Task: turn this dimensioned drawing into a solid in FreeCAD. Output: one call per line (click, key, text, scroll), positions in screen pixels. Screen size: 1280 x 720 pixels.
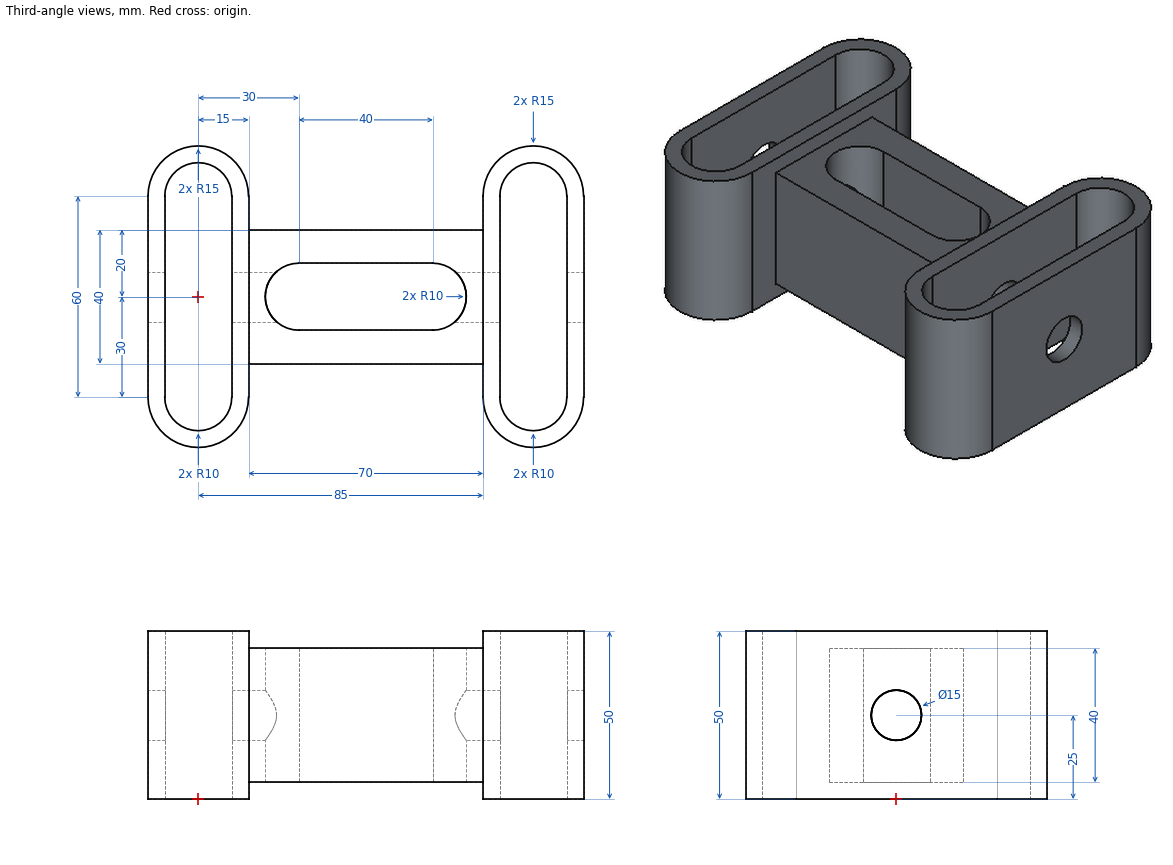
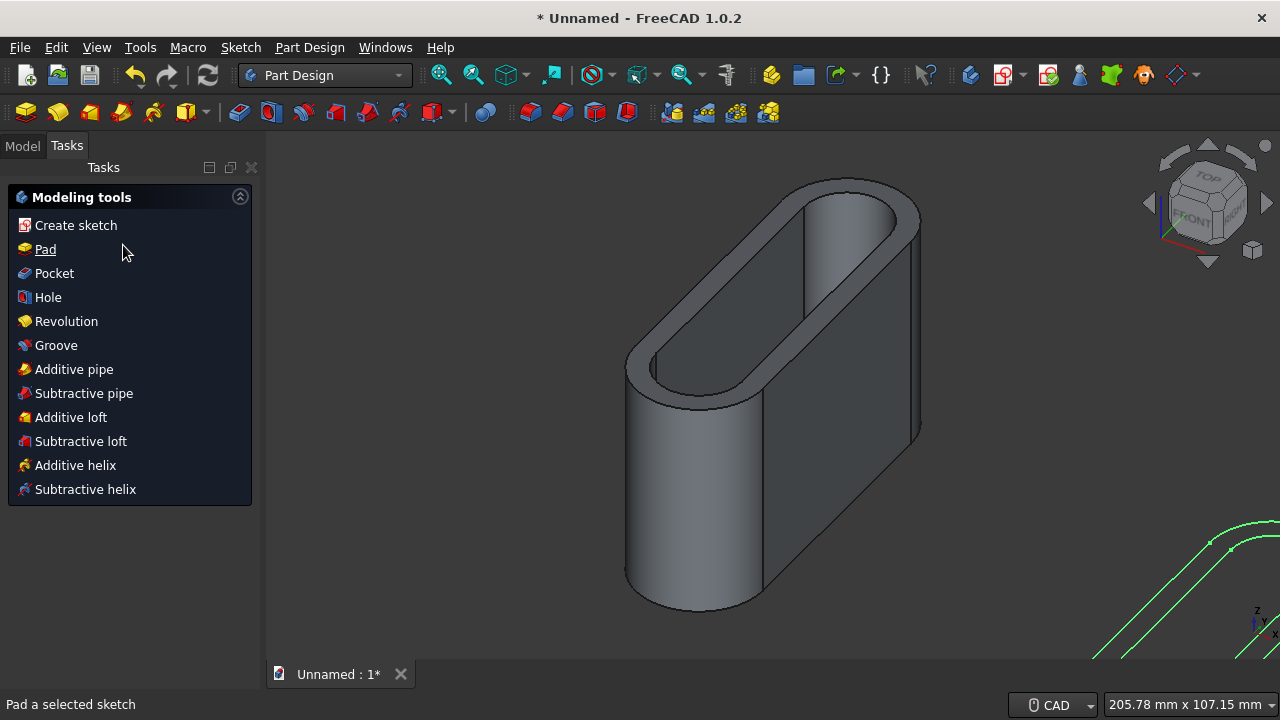
click(26, 112)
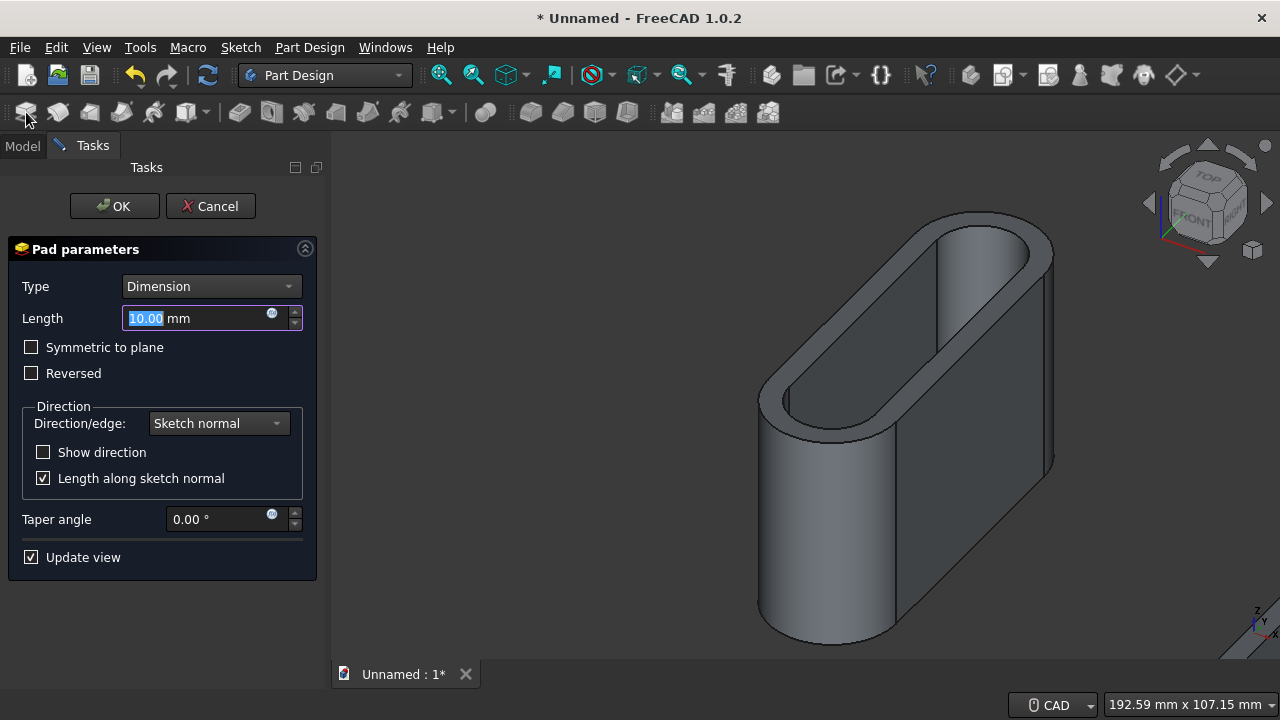
text(50)
key(Tab)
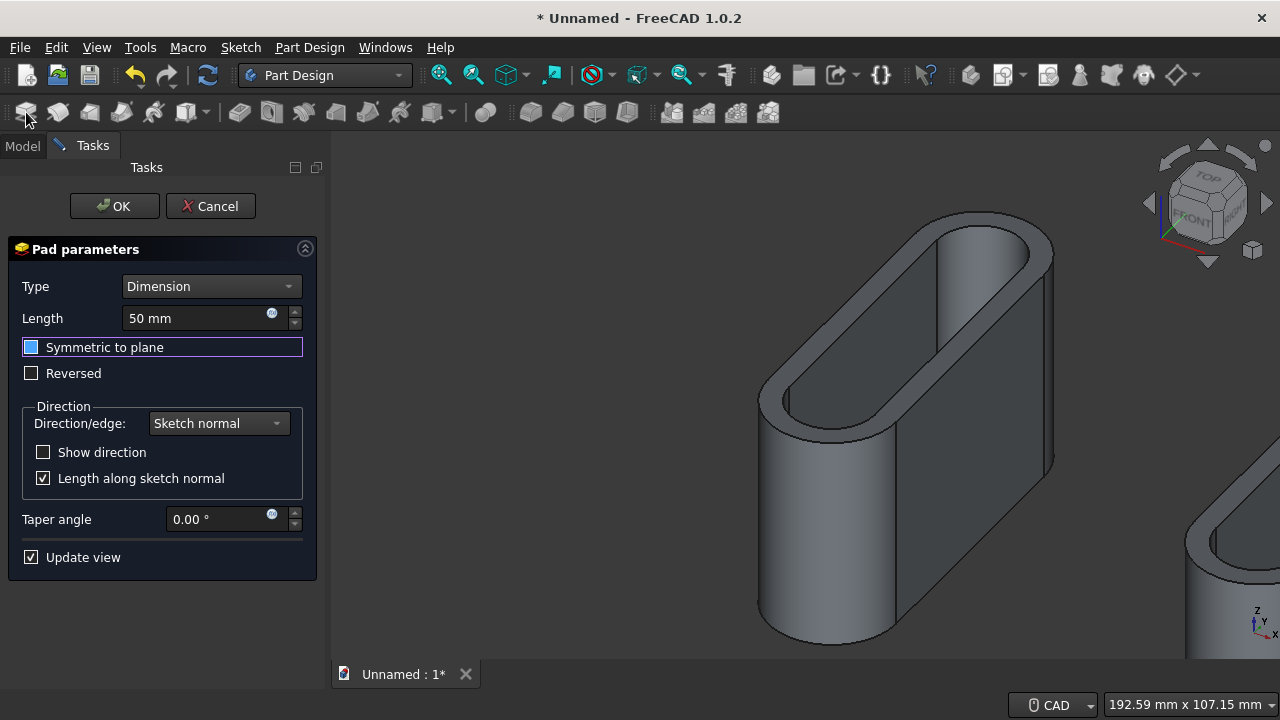
click(115, 206)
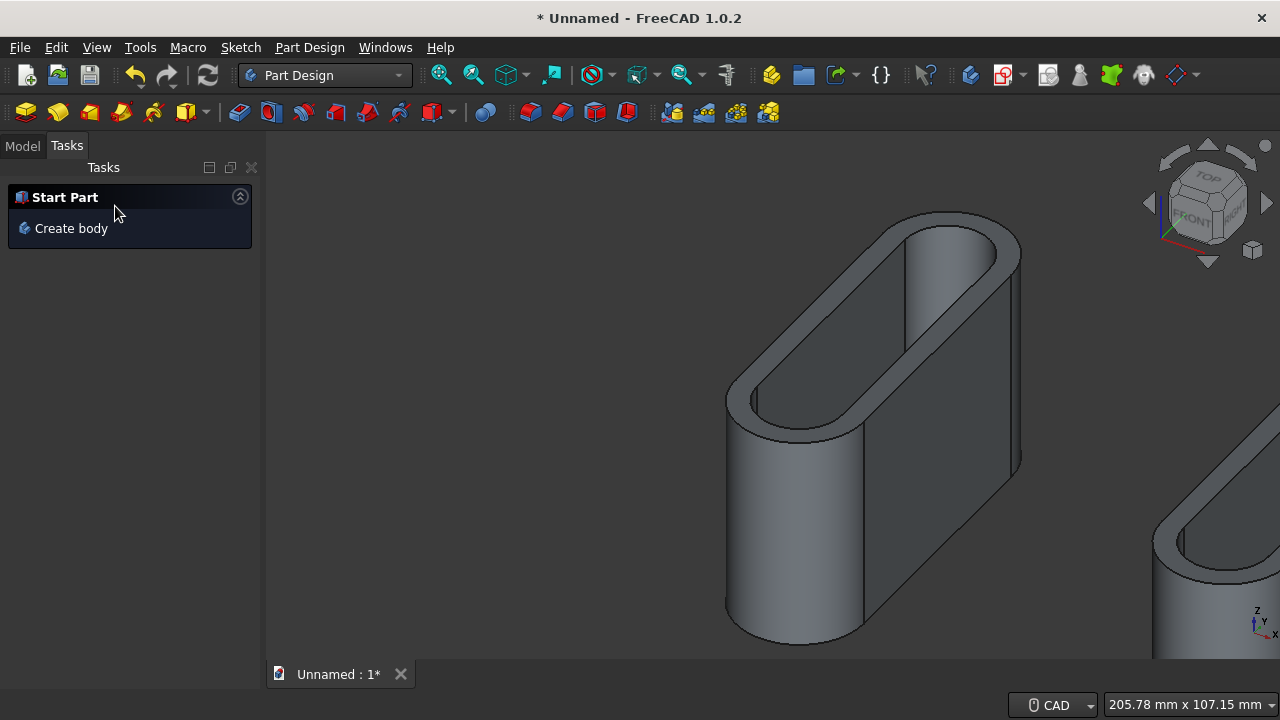
click(442, 76)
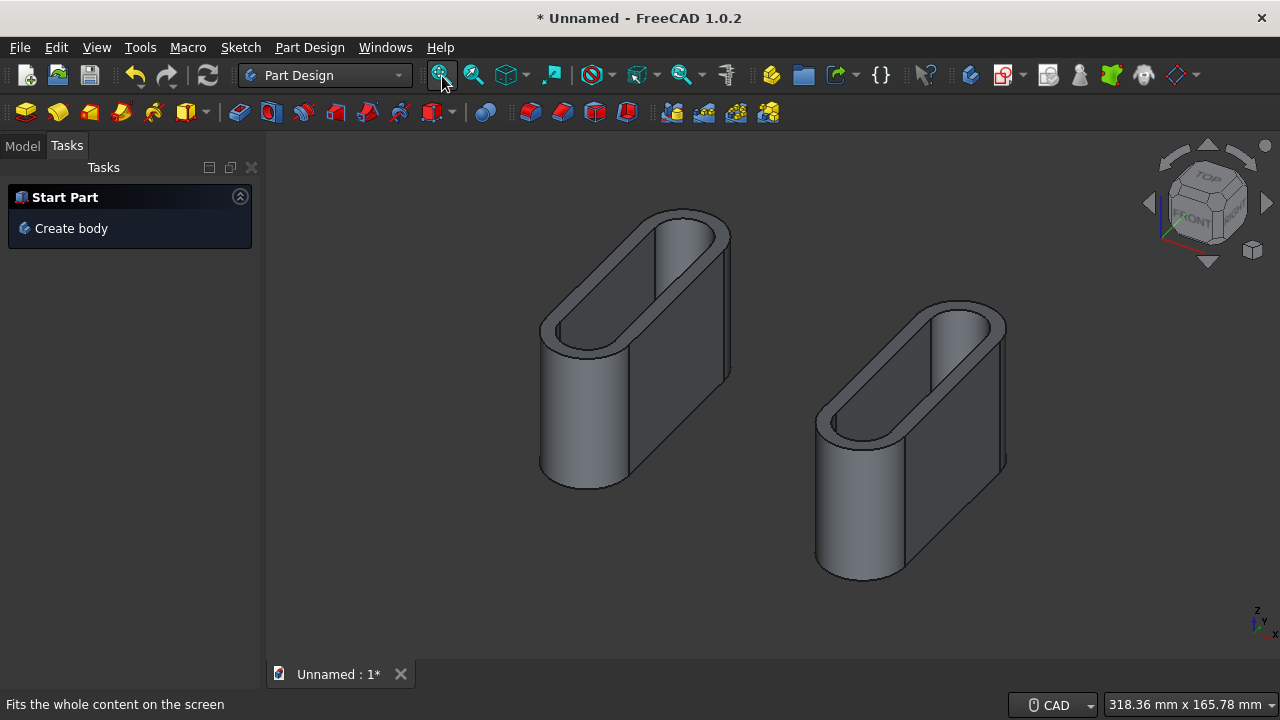
click(23, 145)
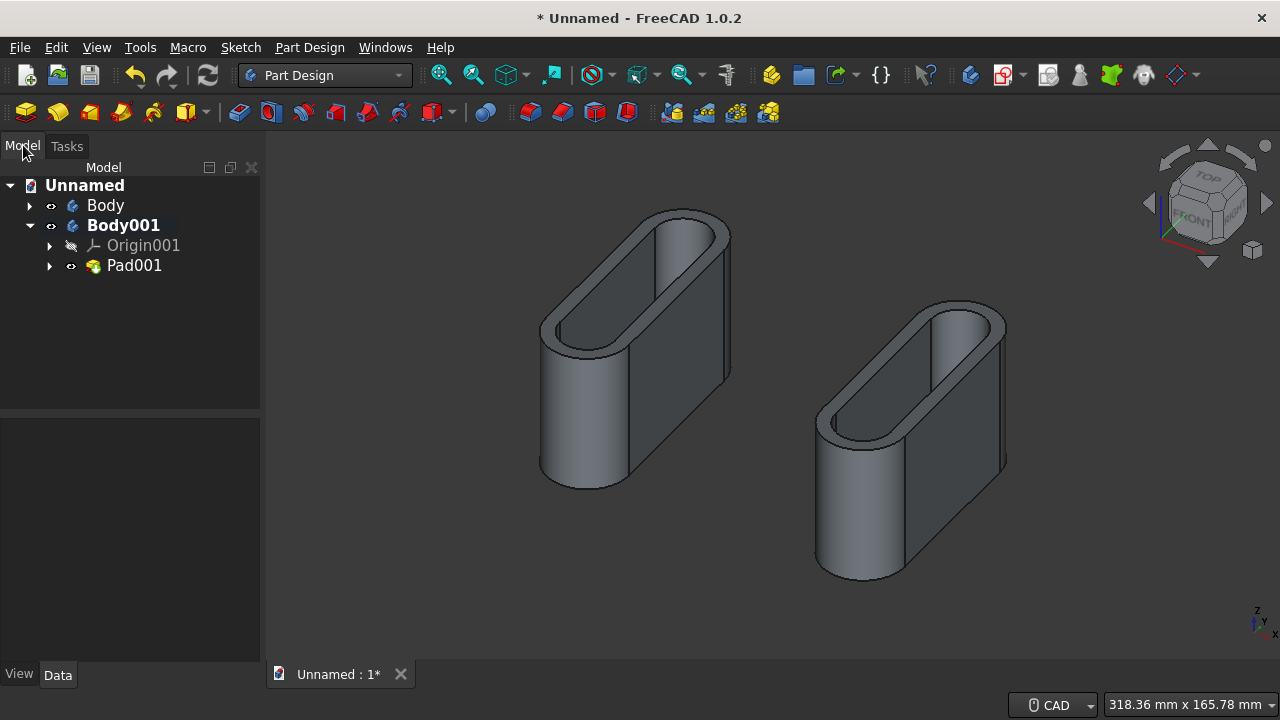
double_click(96, 206)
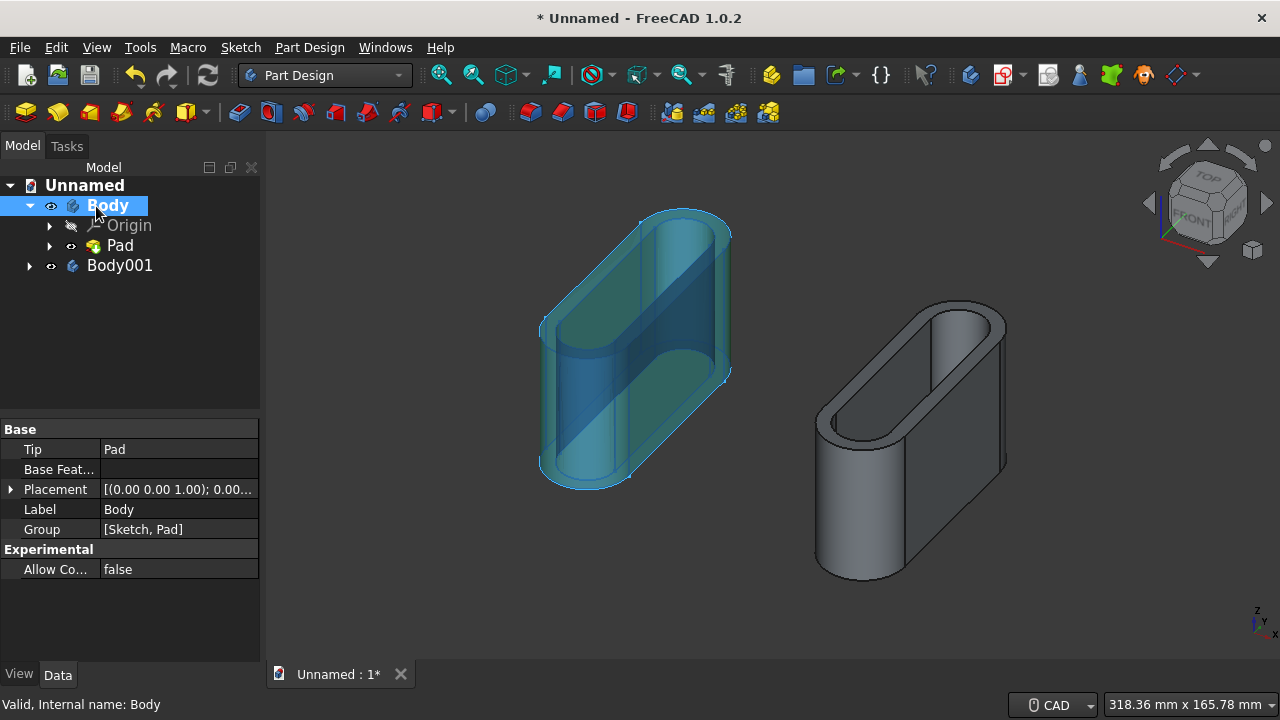
click(96, 206)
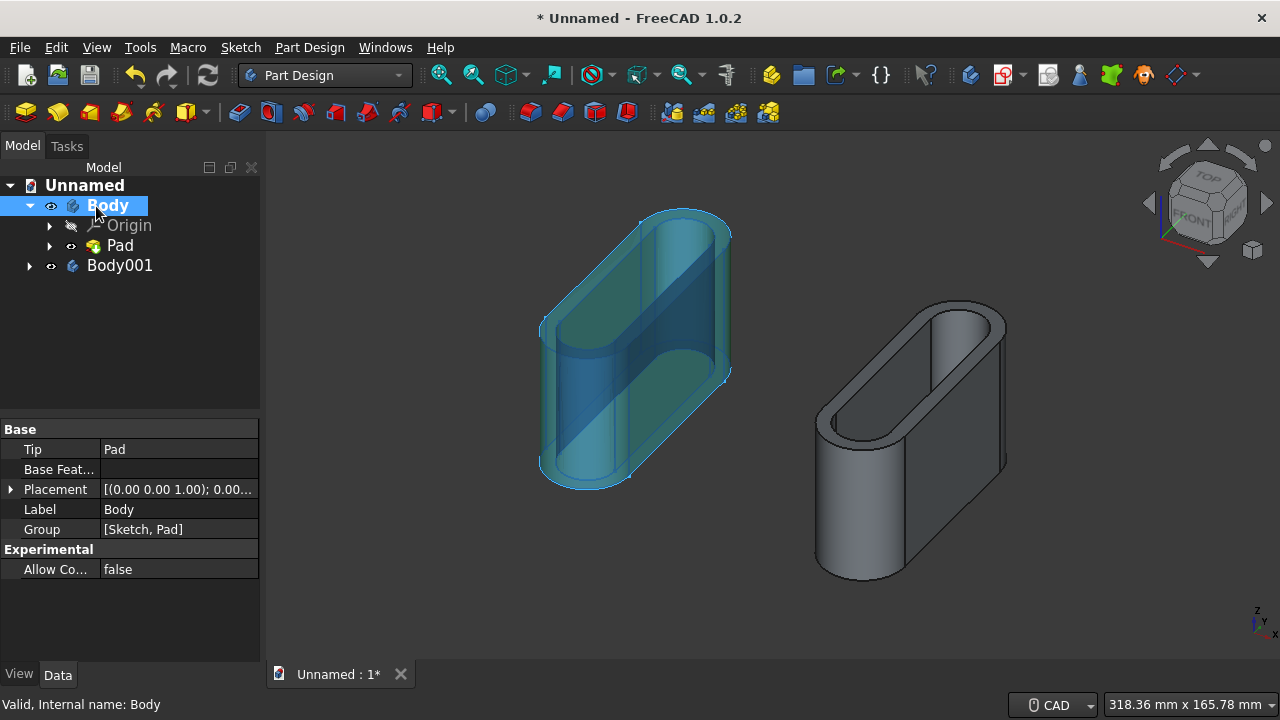
click(146, 569)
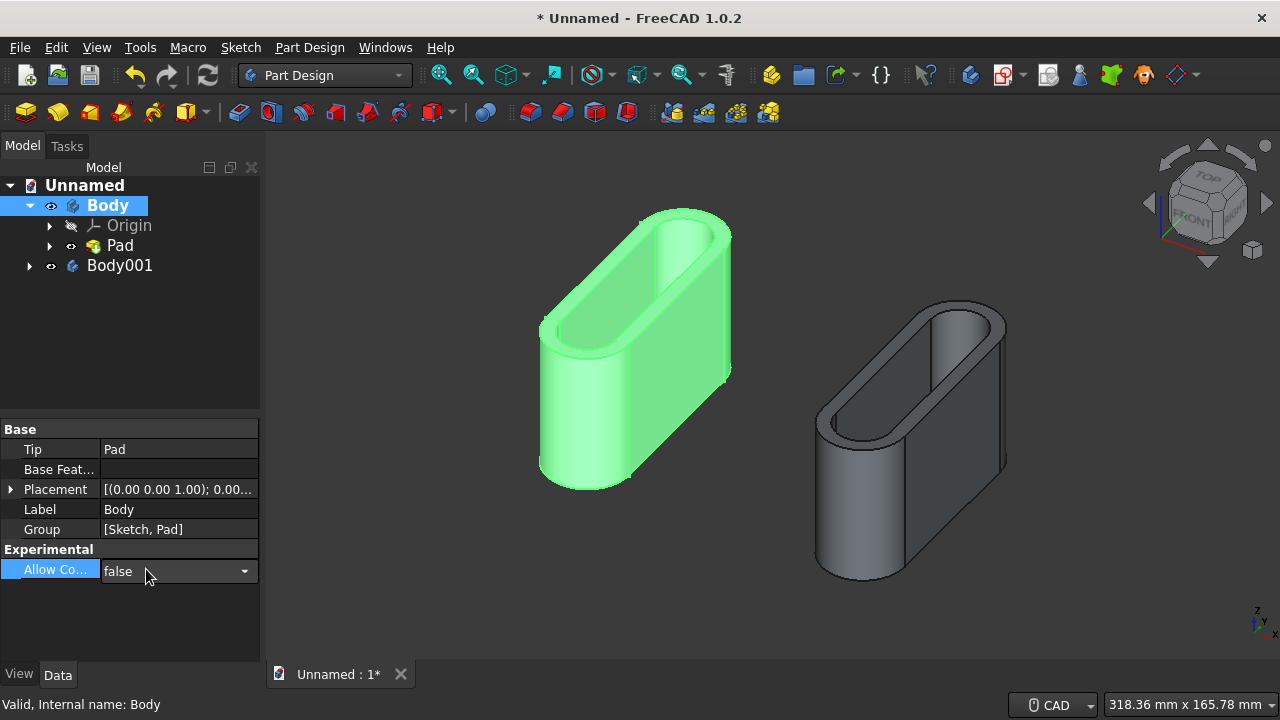
click(146, 569)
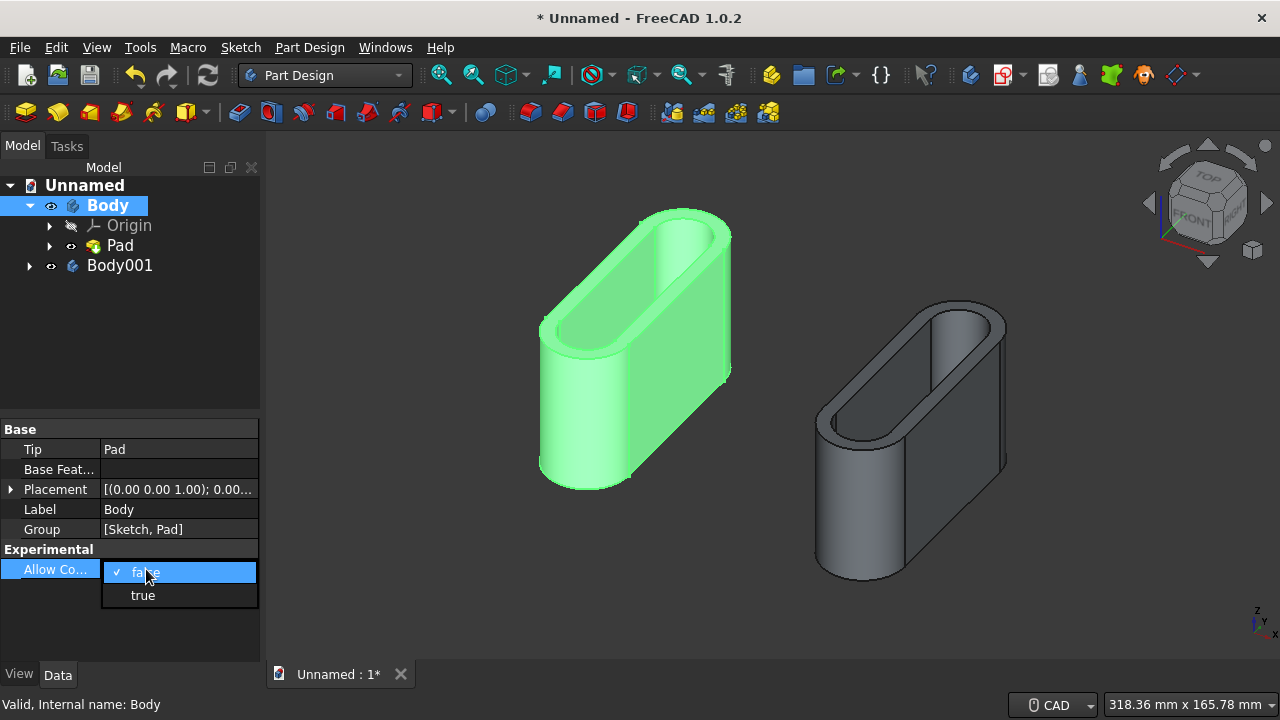
click(179, 596)
key(Return)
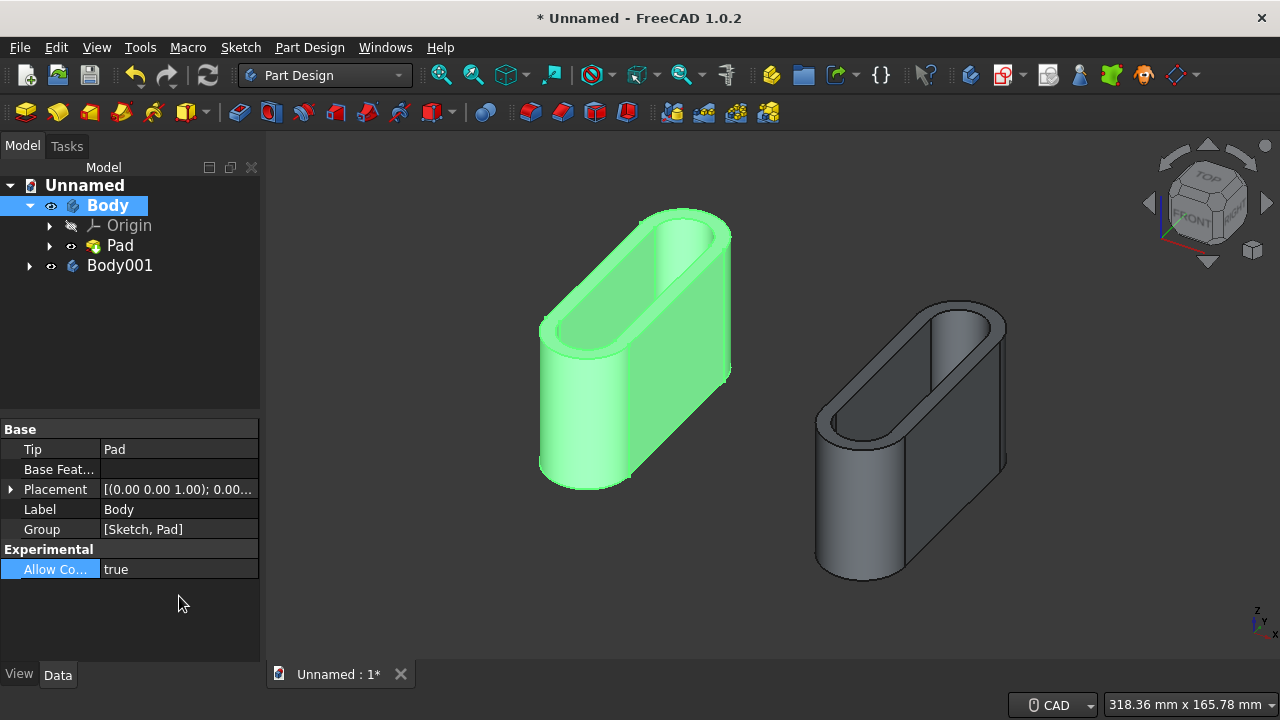
click(96, 266)